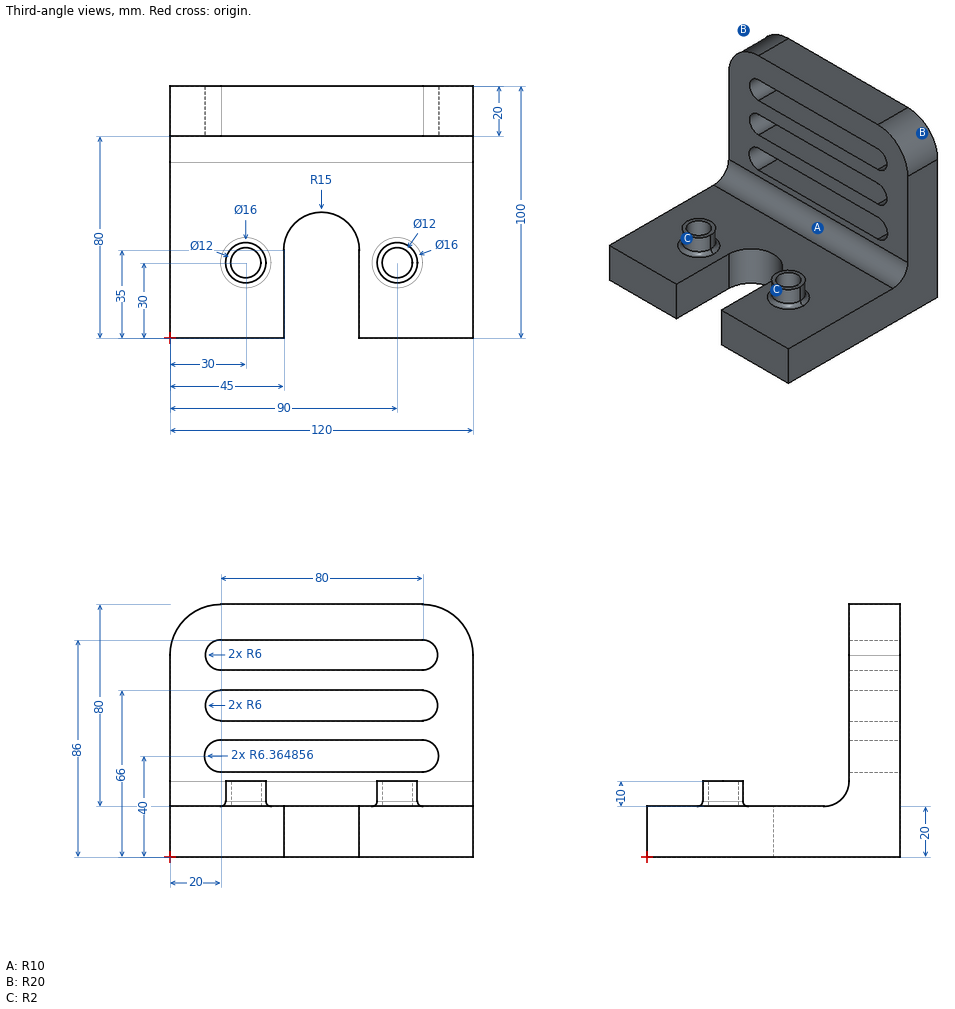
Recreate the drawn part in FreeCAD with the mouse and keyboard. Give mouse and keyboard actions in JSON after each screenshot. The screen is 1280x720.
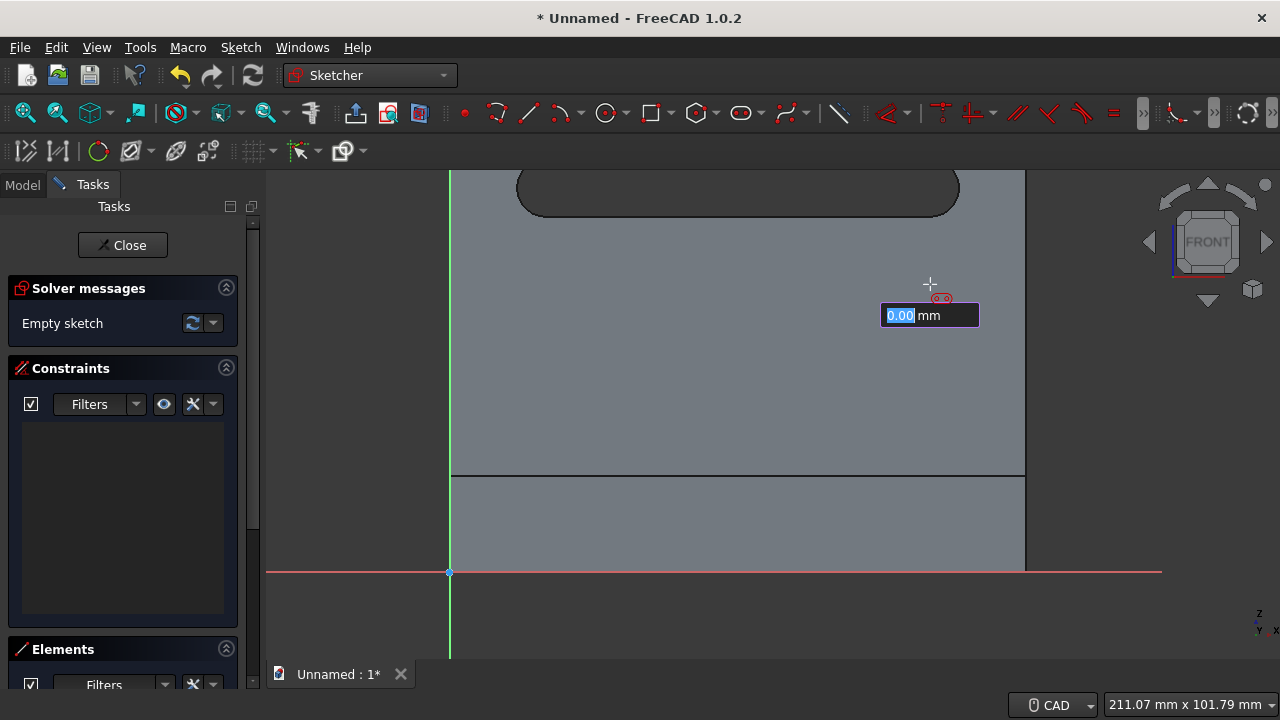
{"action": "left_click", "coordinate": [738, 255]}
{"action": "key", "text": "Escape"}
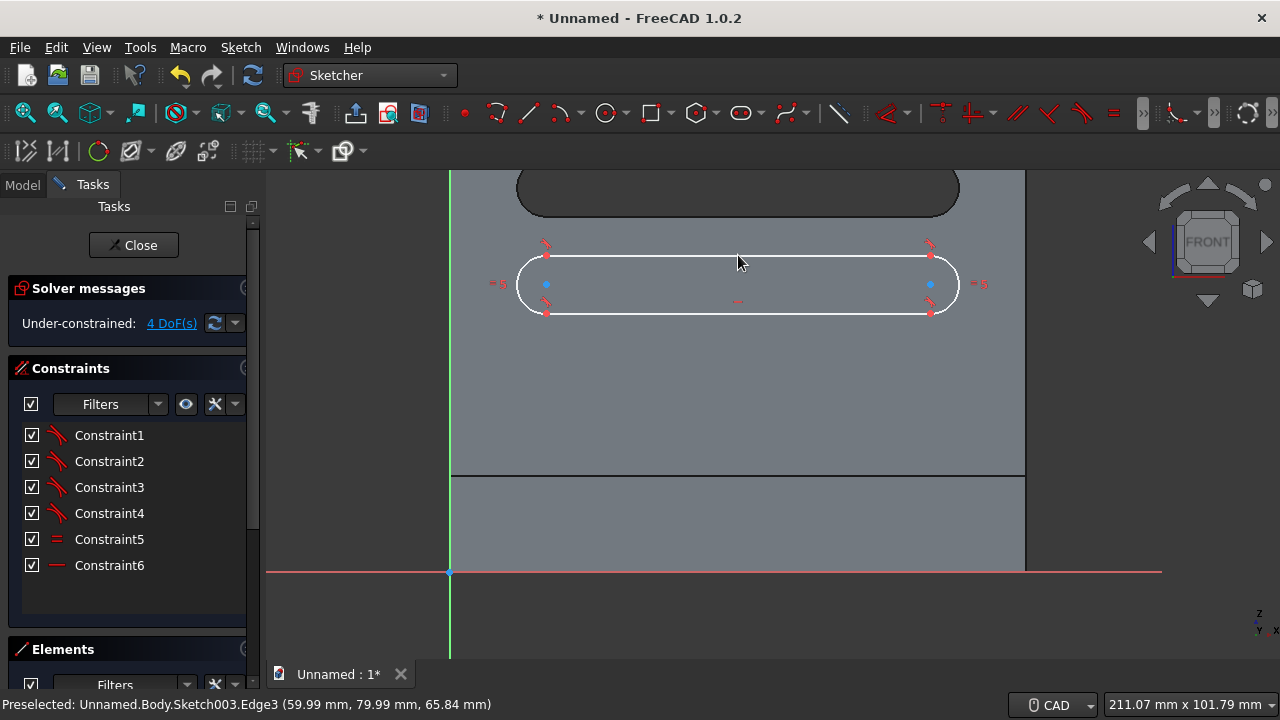
{"action": "left_click", "coordinate": [886, 114]}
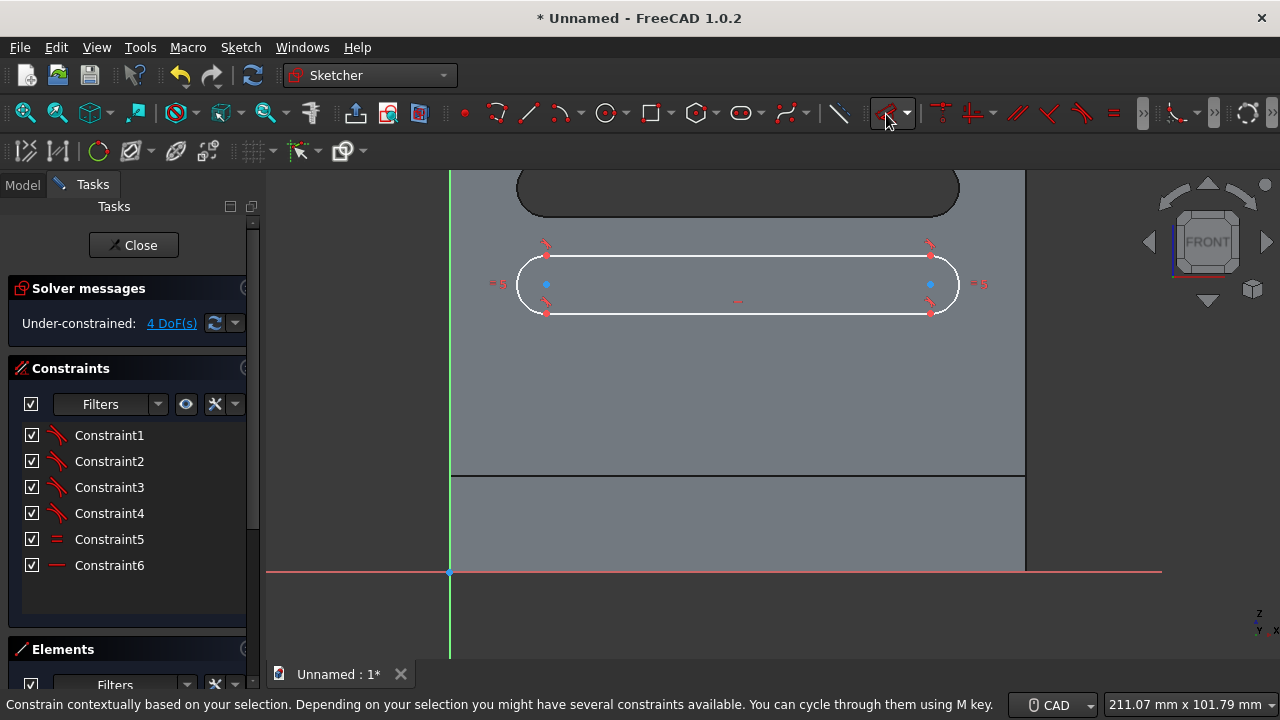
{"action": "scroll", "coordinate": [523, 268], "scroll_direction": "up", "scroll_amount": 2}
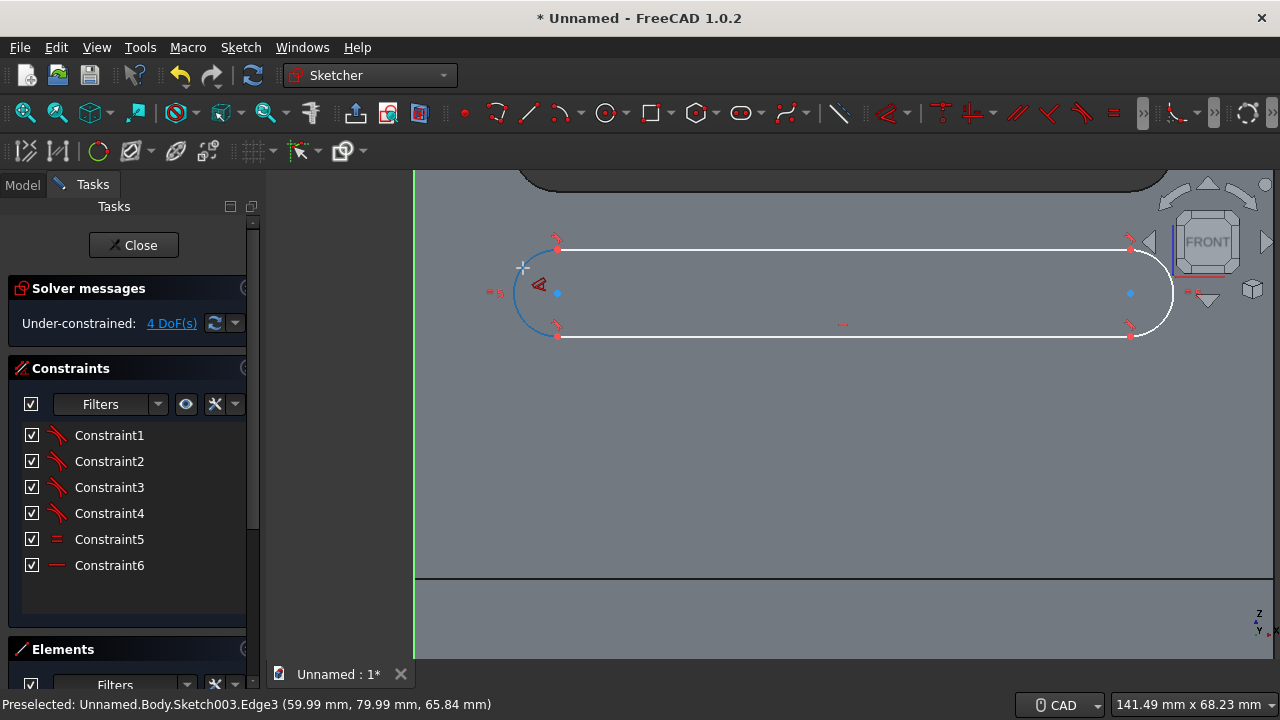
{"action": "left_click", "coordinate": [522, 268]}
{"action": "left_click", "coordinate": [496, 249]}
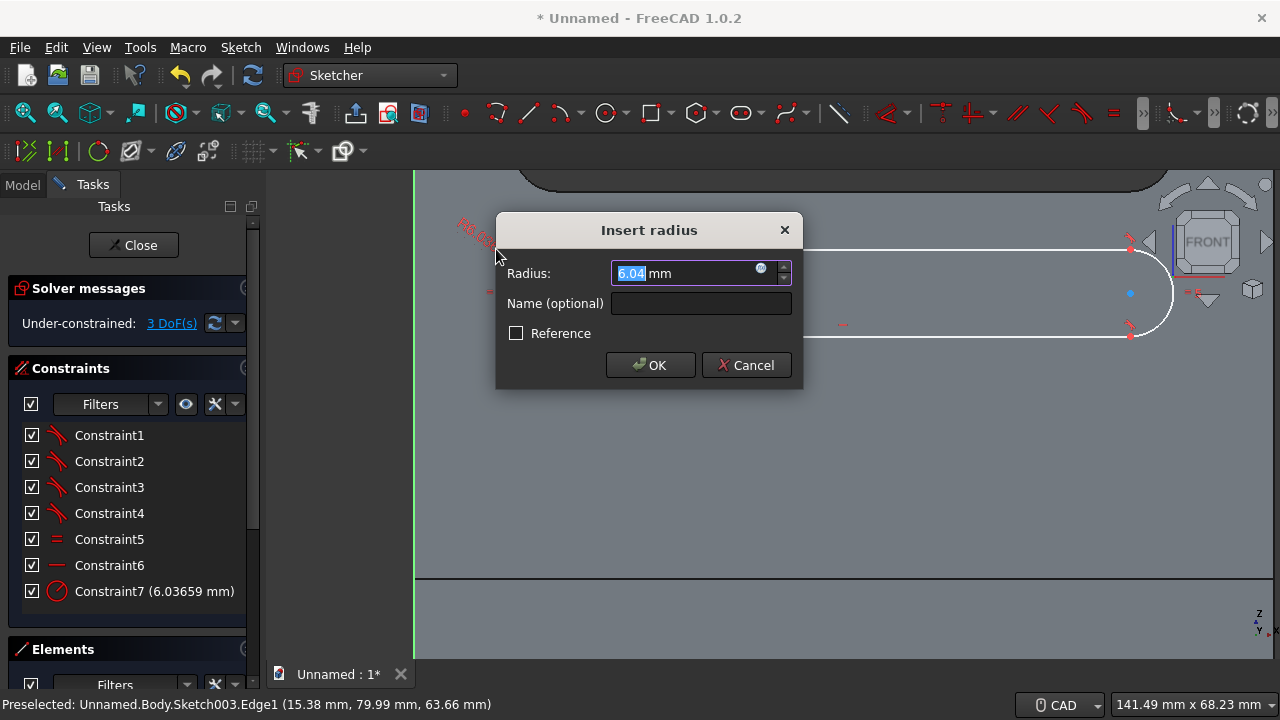
{"action": "type", "text": "6"}
{"action": "key", "text": "Return"}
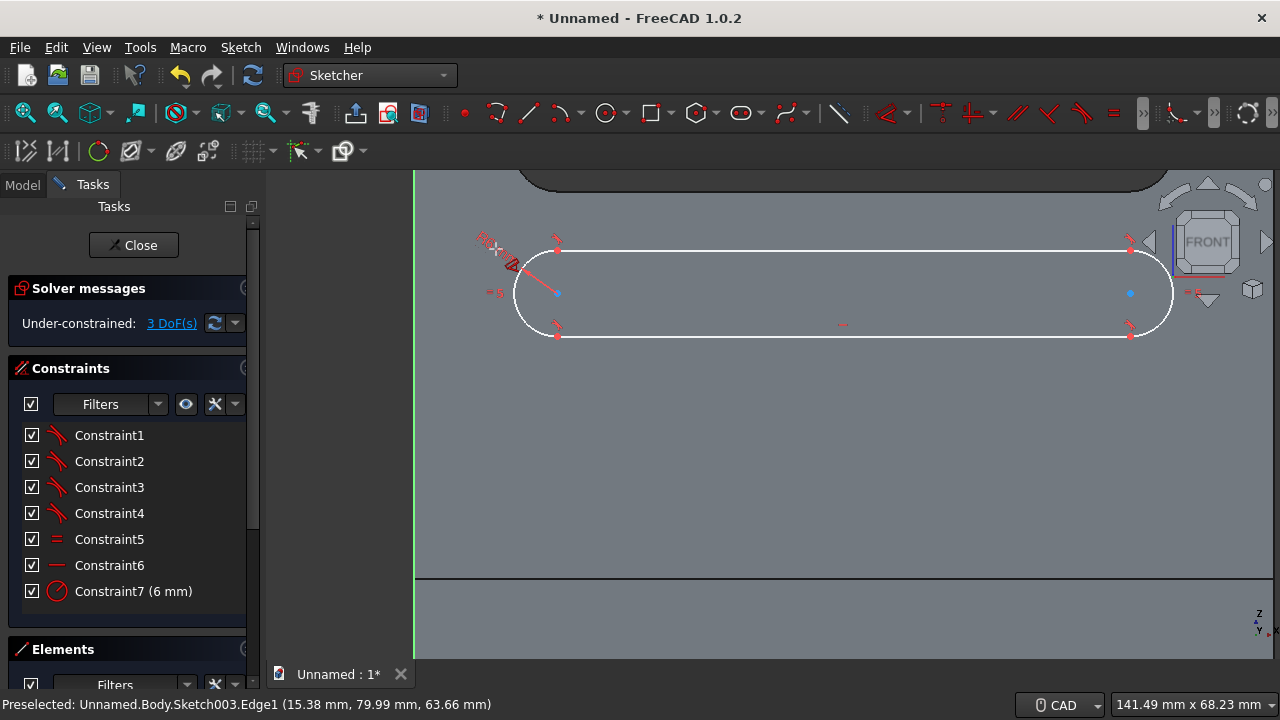
{"action": "left_click", "coordinate": [729, 251]}
{"action": "left_click", "coordinate": [836, 217]}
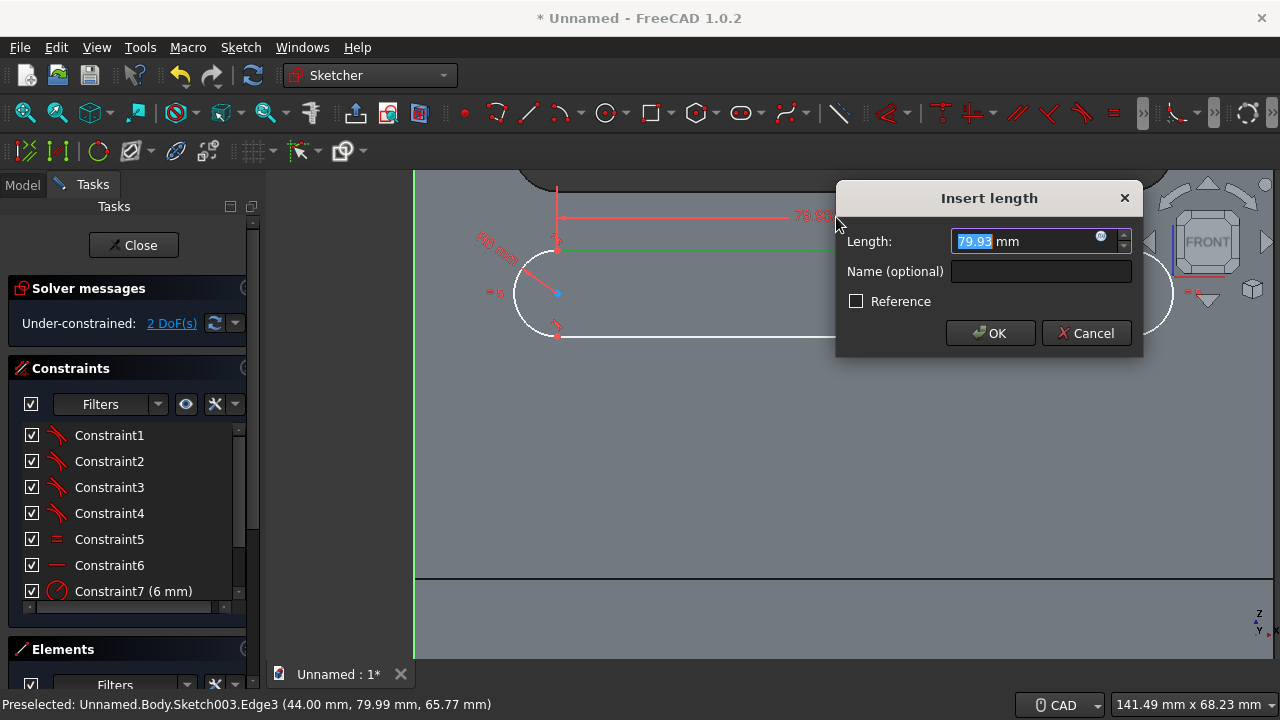
{"action": "type", "text": "80"}
{"action": "key", "text": "Return"}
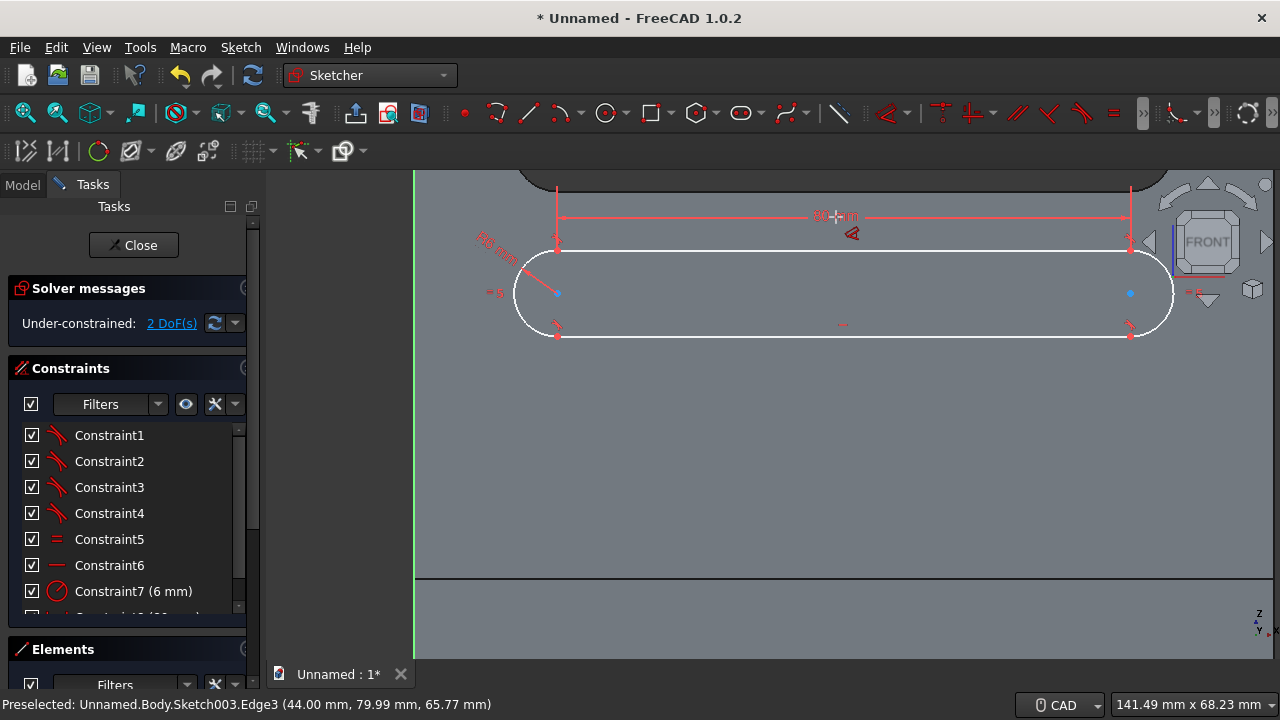
{"action": "left_click", "coordinate": [557, 251]}
{"action": "left_click", "coordinate": [485, 217]}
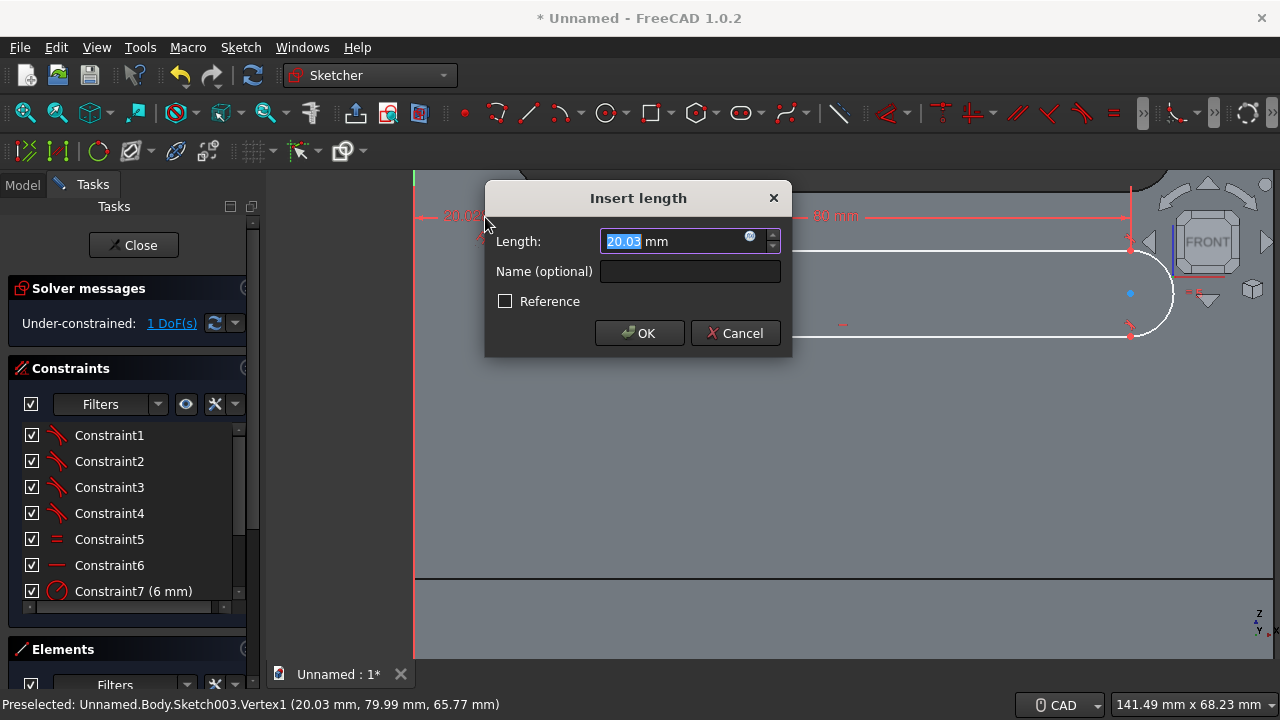
{"action": "type", "text": "20"}
{"action": "key", "text": "Return"}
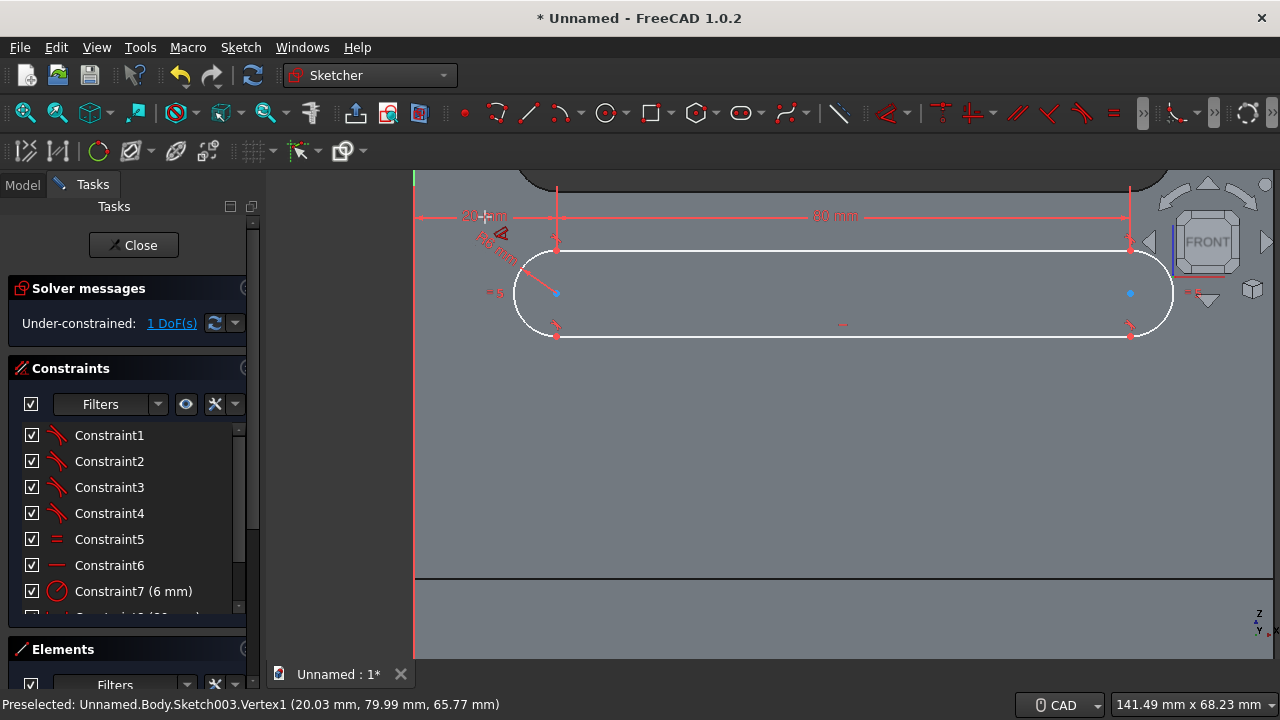
{"action": "left_click", "coordinate": [557, 251]}
{"action": "left_click", "coordinate": [380, 441]}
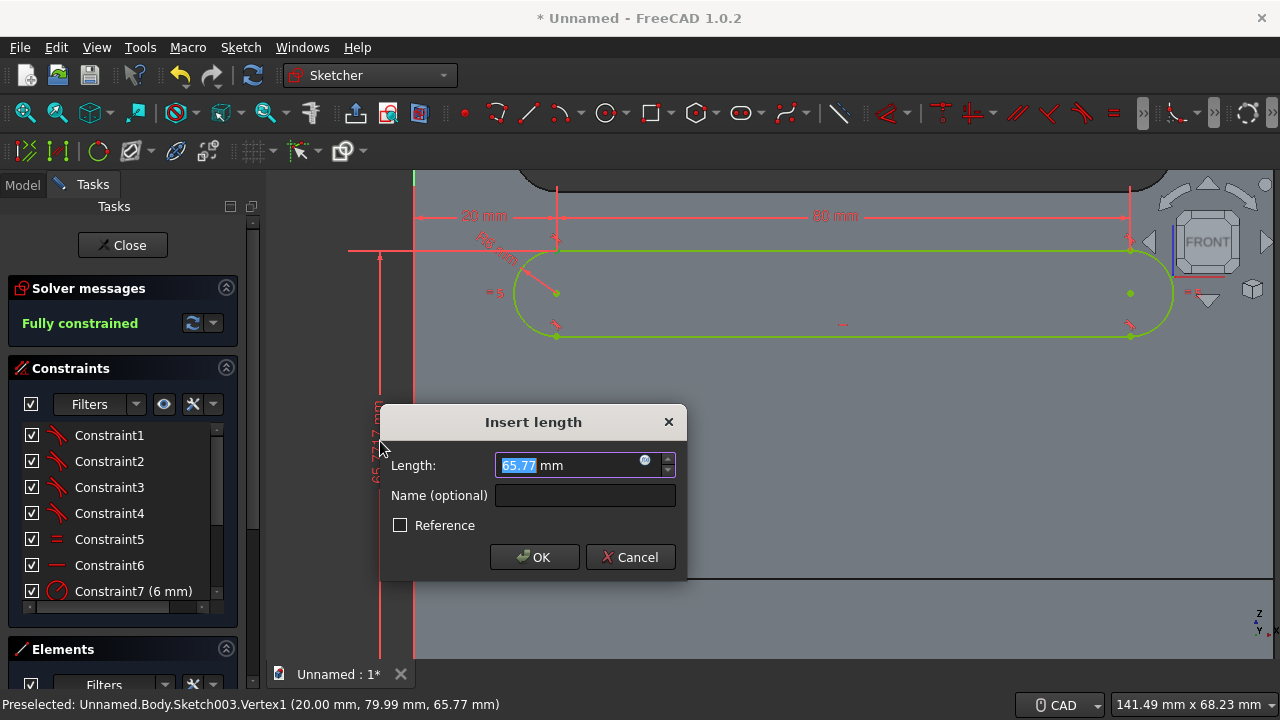
{"action": "type", "text": "66"}
{"action": "key", "text": "Return"}
{"action": "key", "text": "Escape"}